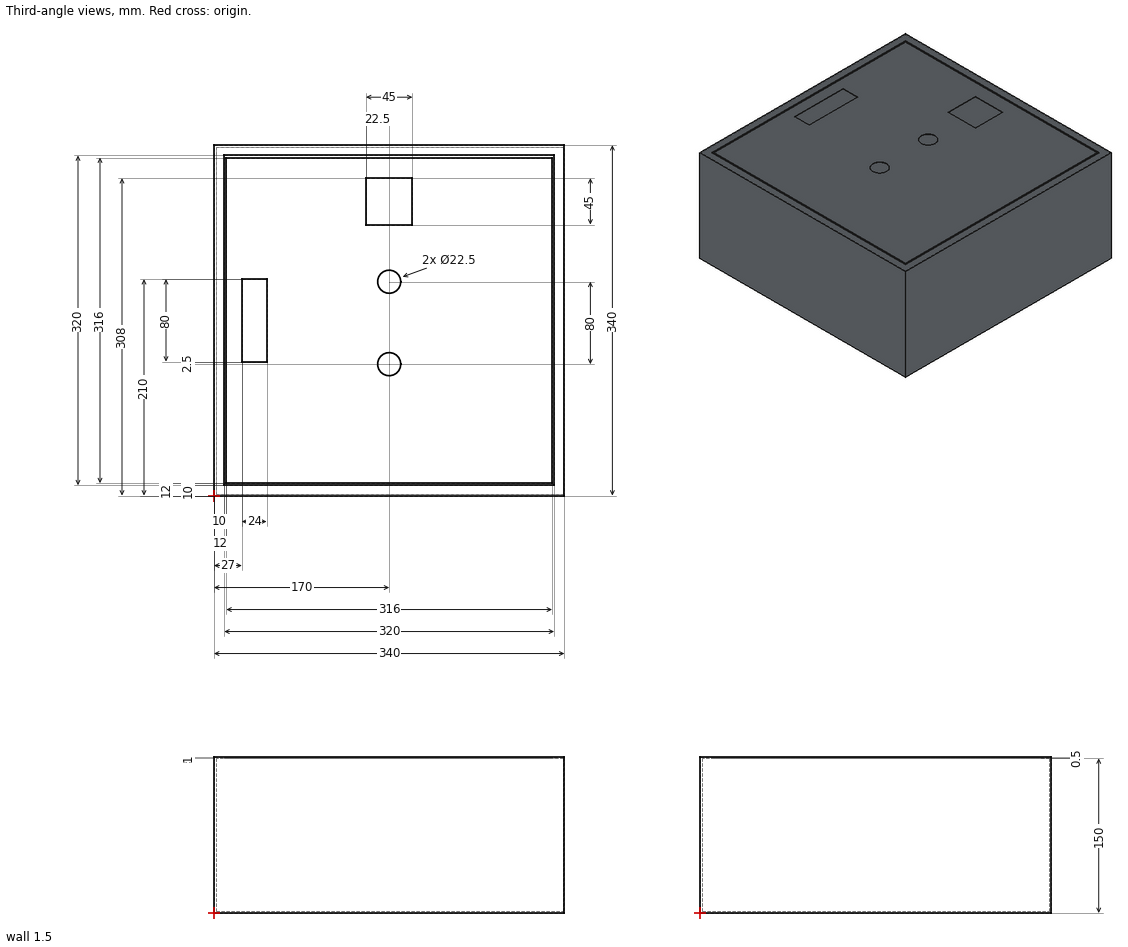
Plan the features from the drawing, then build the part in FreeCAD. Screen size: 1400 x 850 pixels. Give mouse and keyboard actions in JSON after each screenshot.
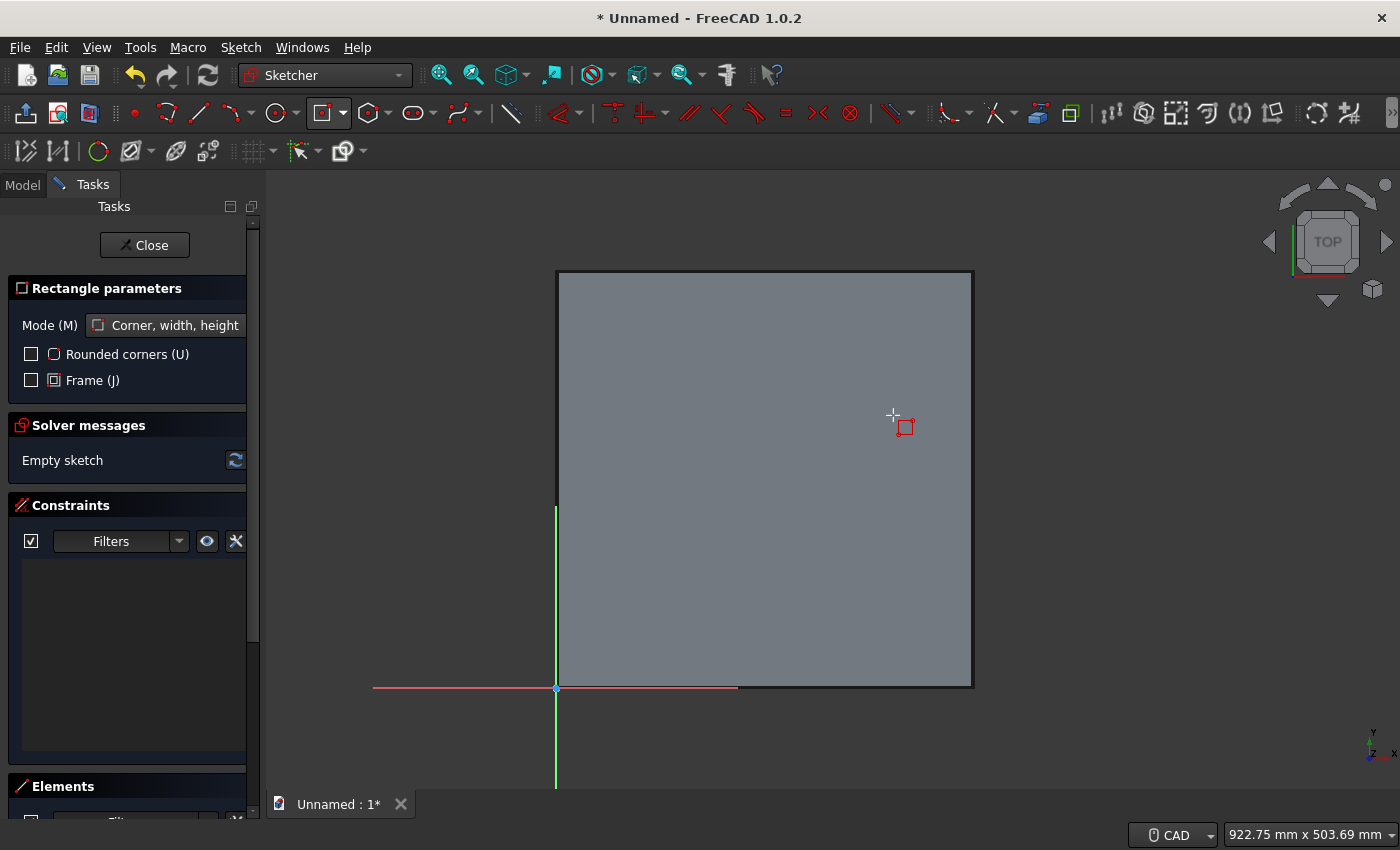
{"action": "left_click", "coordinate": [556, 688]}
{"action": "mouse_move", "coordinate": [974, 271]}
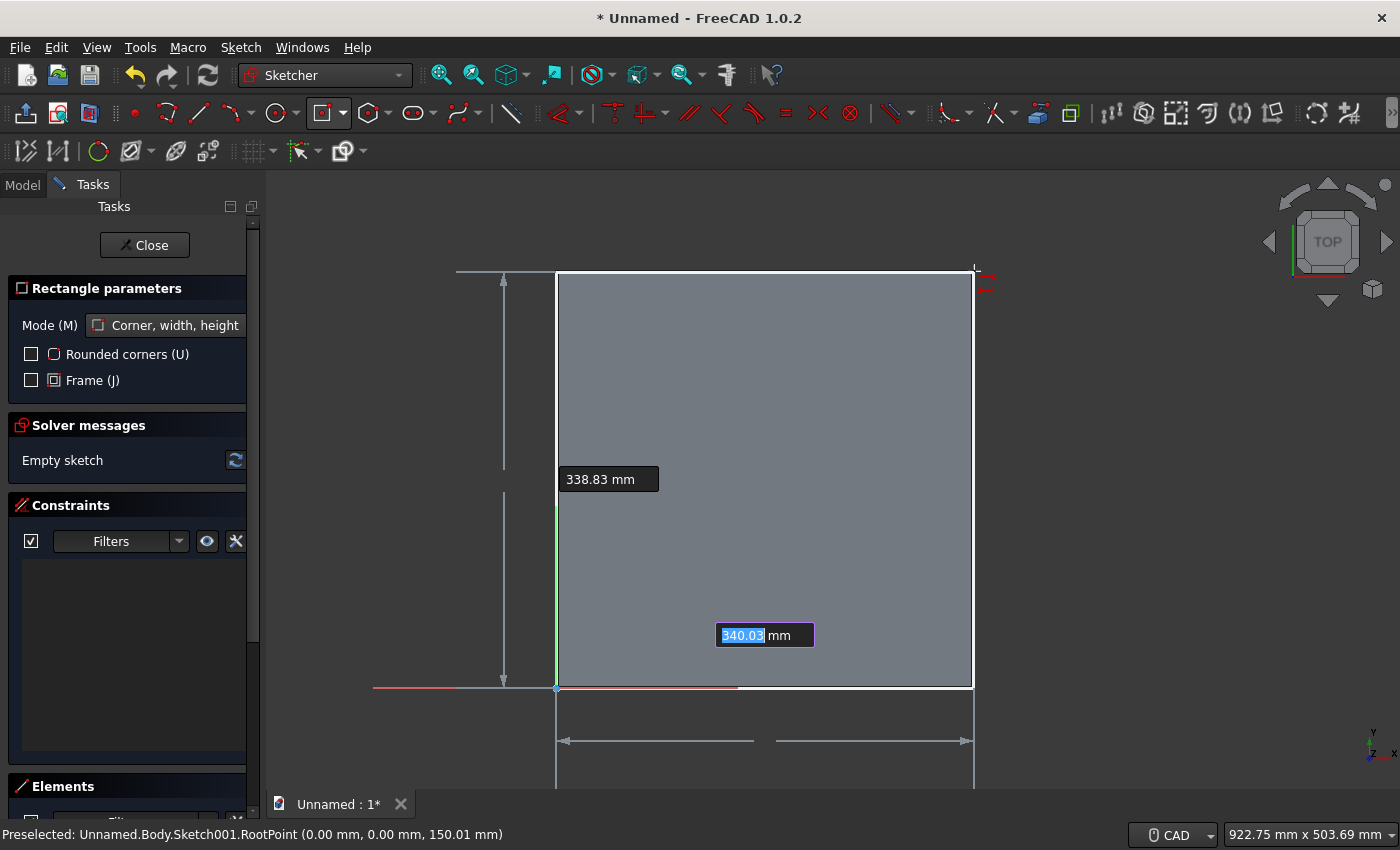
{"action": "type", "text": "340"}
{"action": "key", "text": "Tab"}
{"action": "type", "text": "340"}
{"action": "key", "text": "Return"}
{"action": "key", "text": "Escape"}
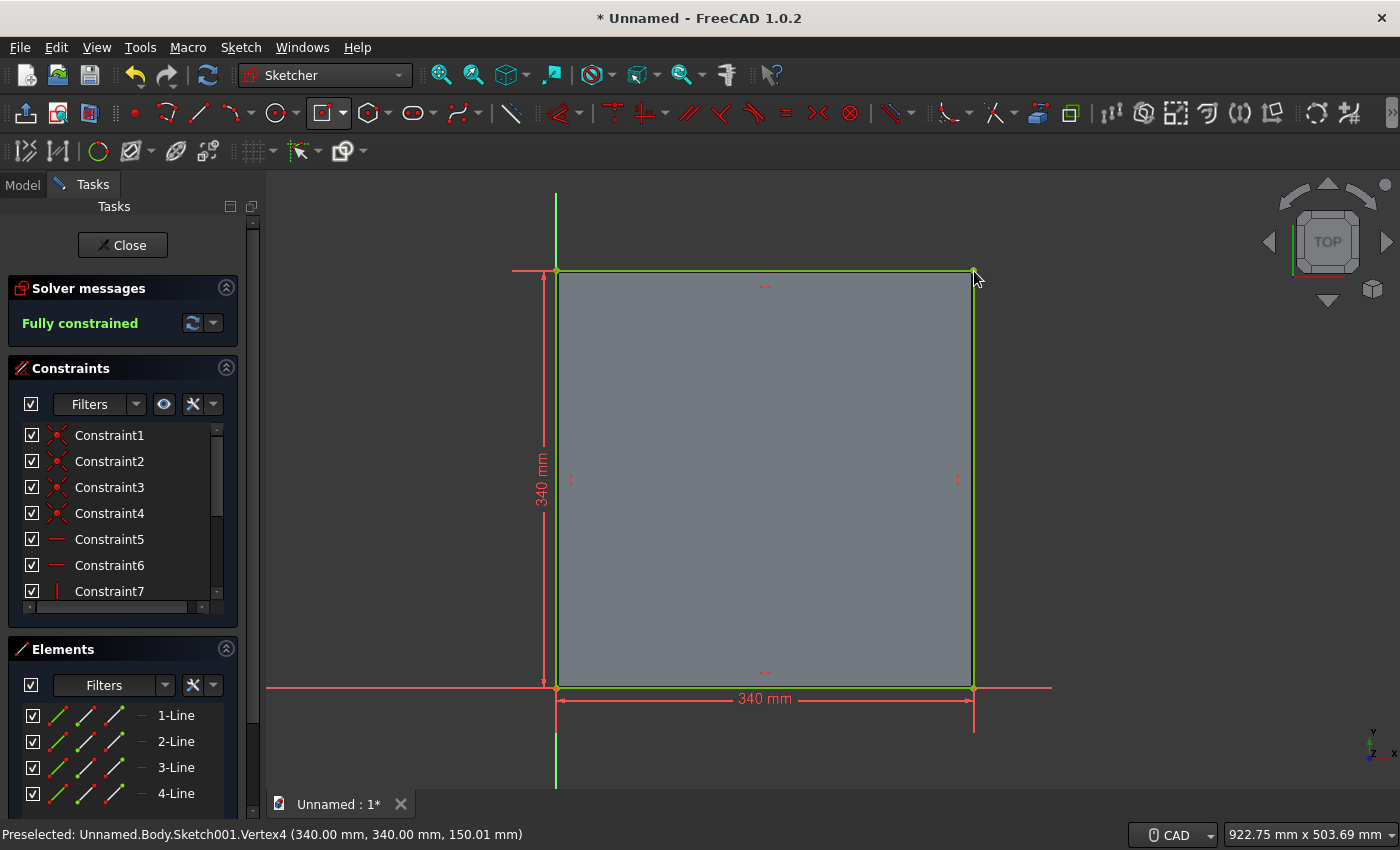
{"action": "left_click", "coordinate": [123, 245]}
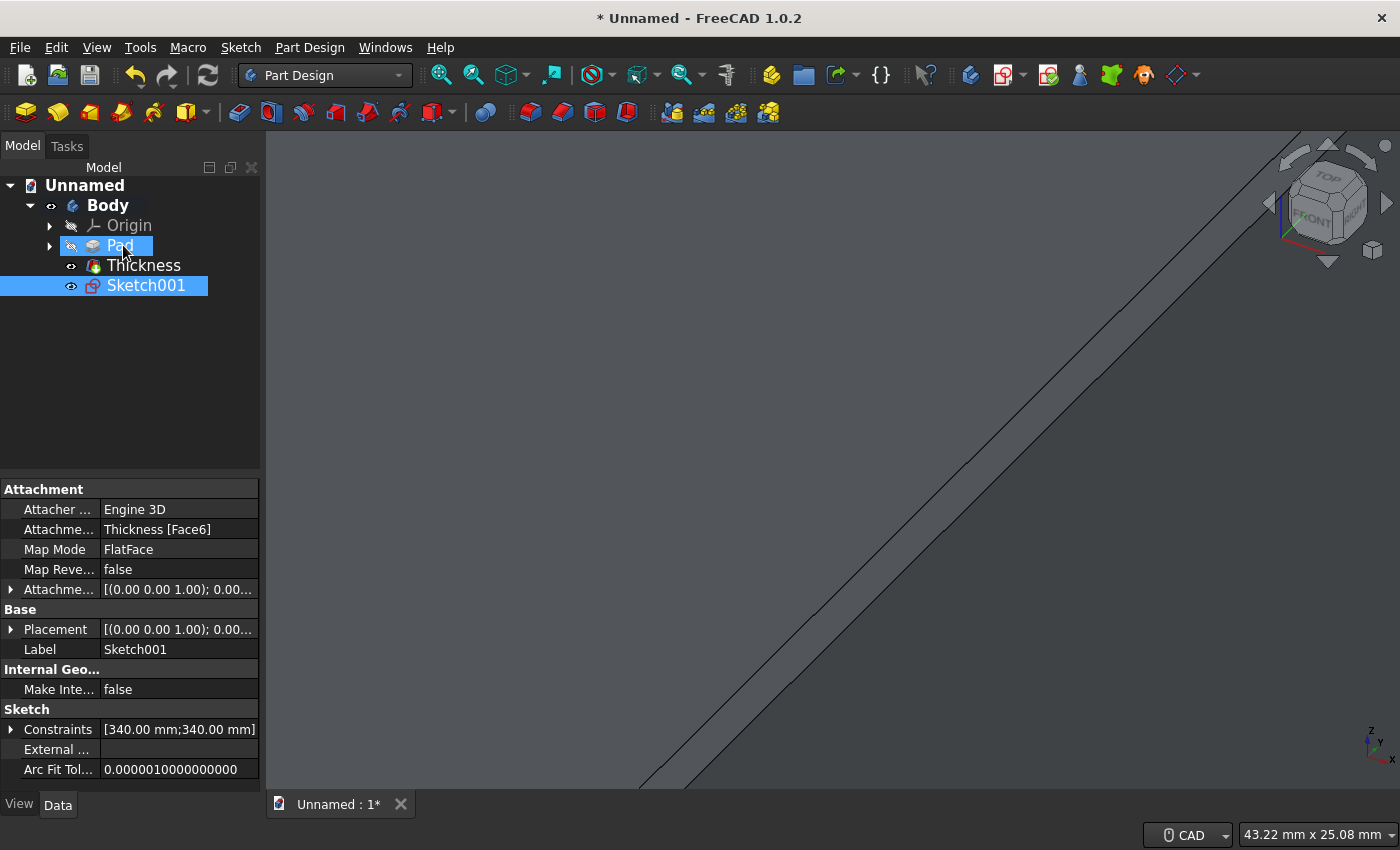
{"action": "left_click", "coordinate": [26, 112]}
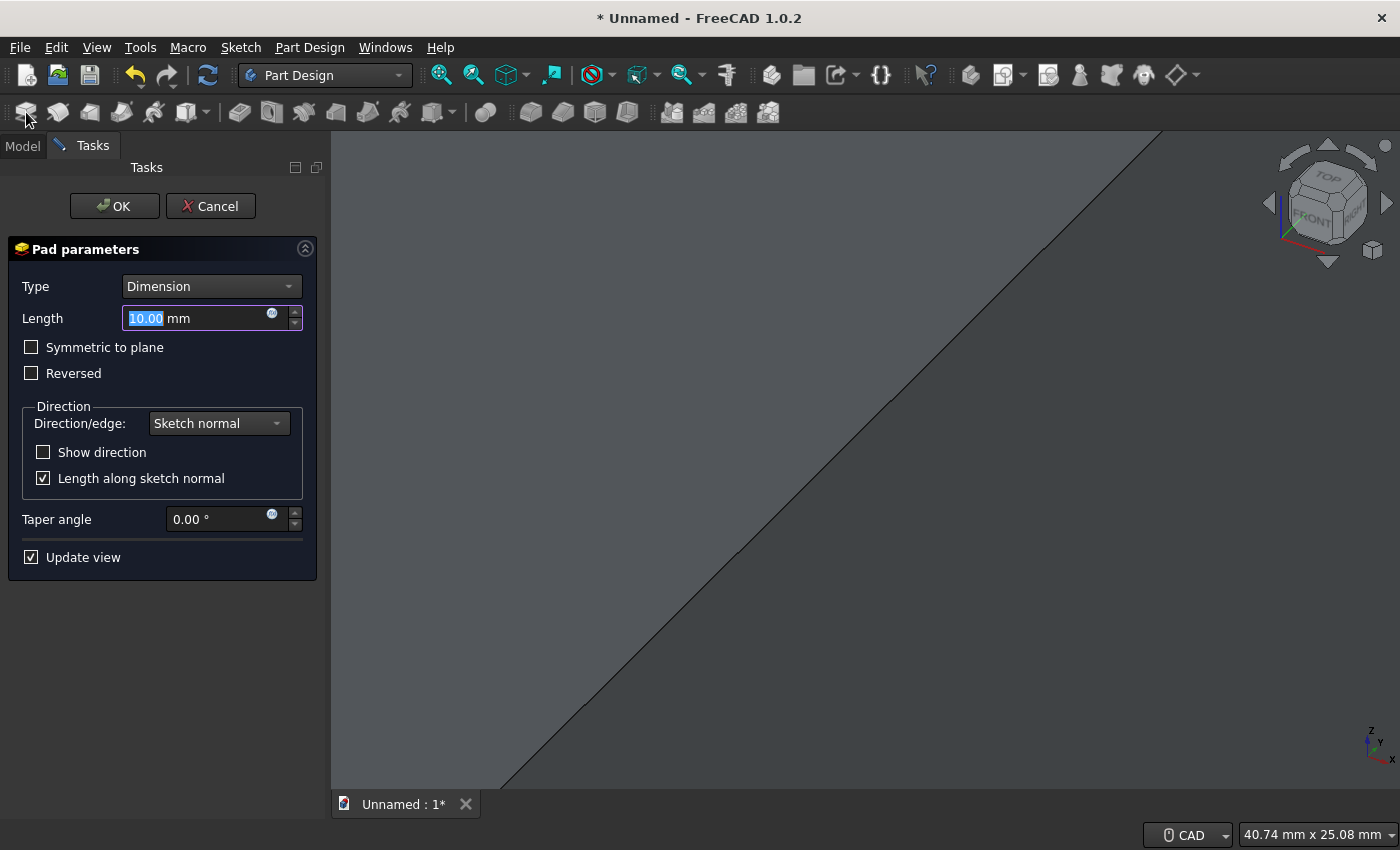
{"action": "type", "text": "1"}
{"action": "key", "text": "Tab"}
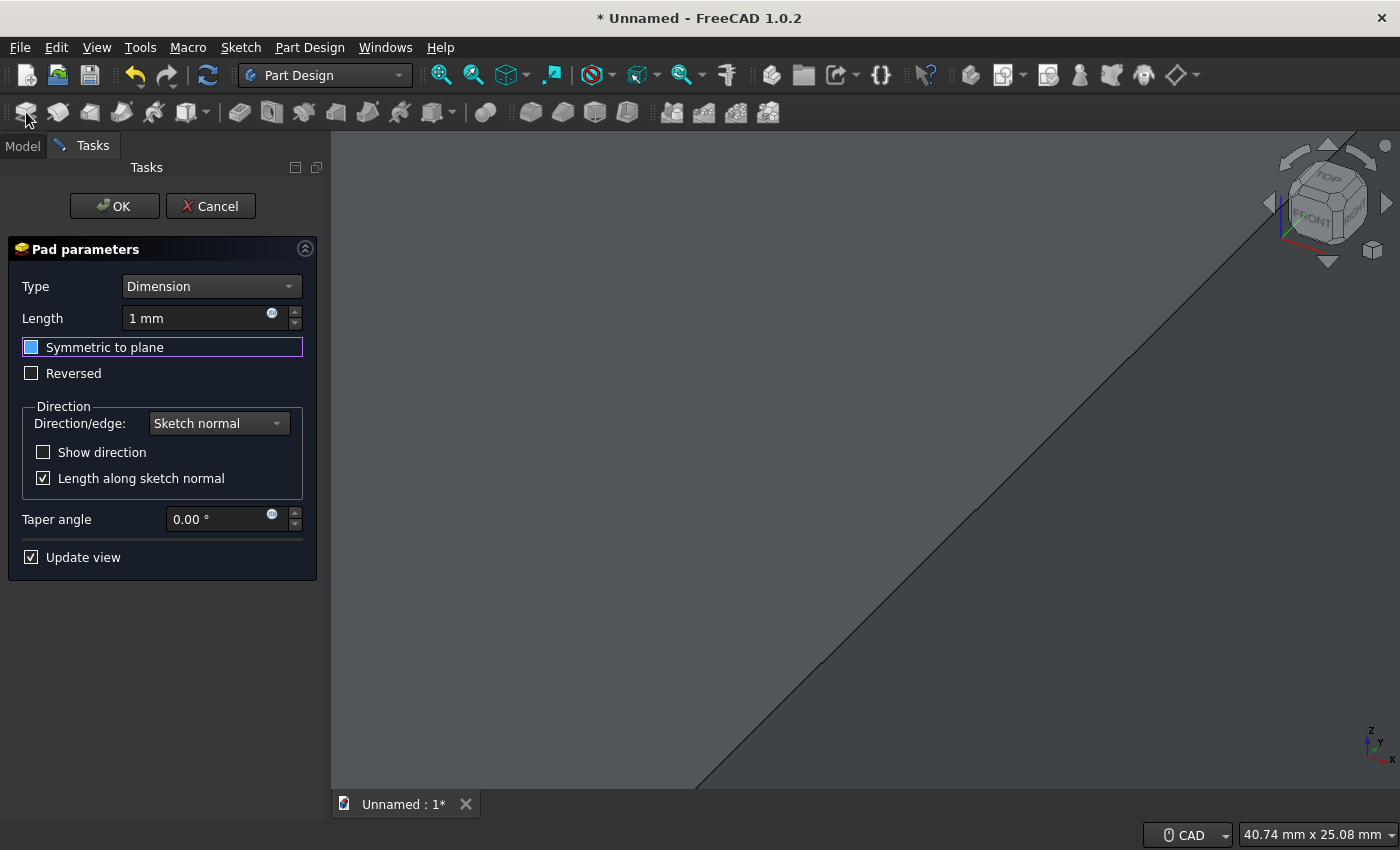
{"action": "left_click", "coordinate": [115, 206]}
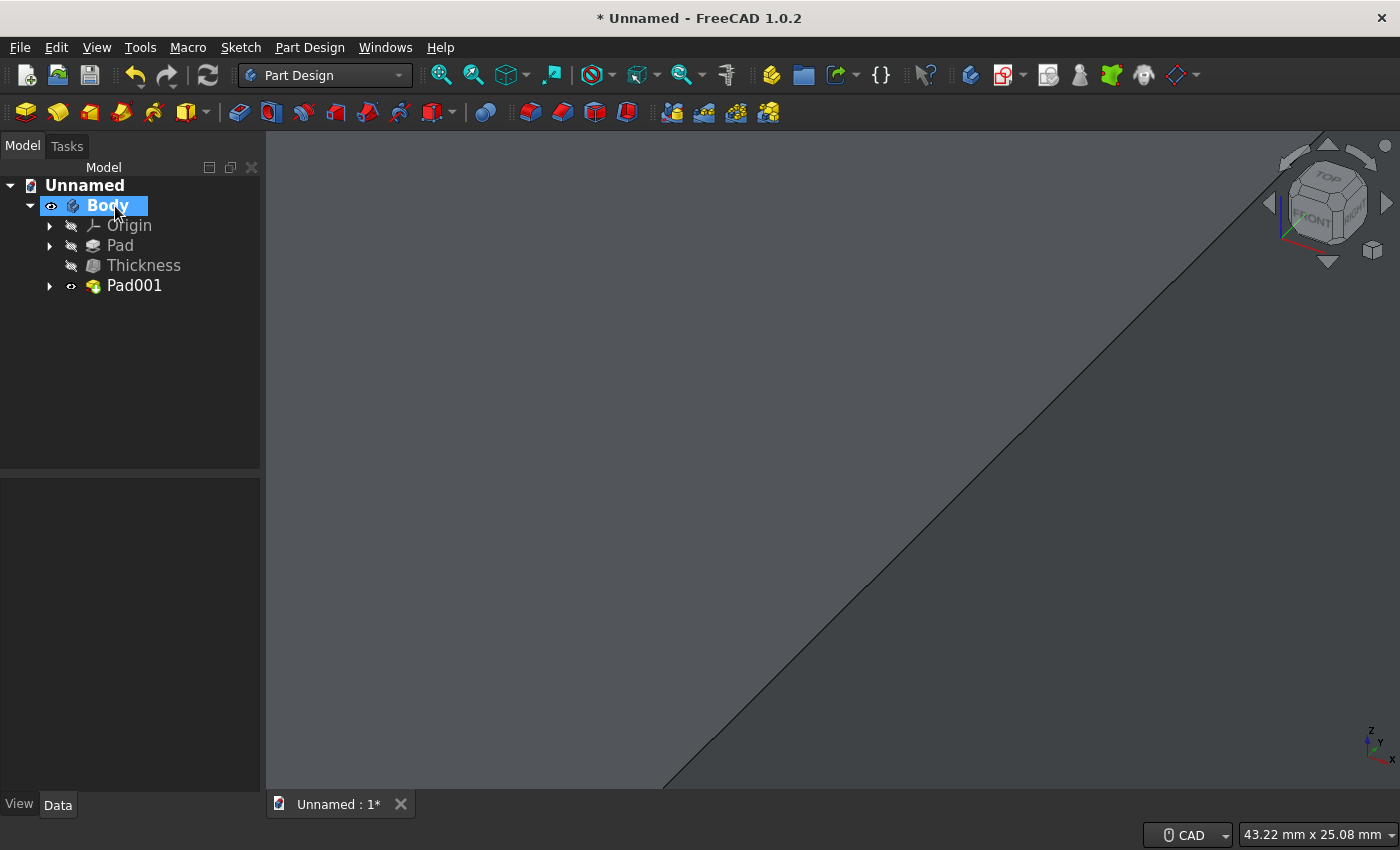
{"action": "key", "text": "v f"}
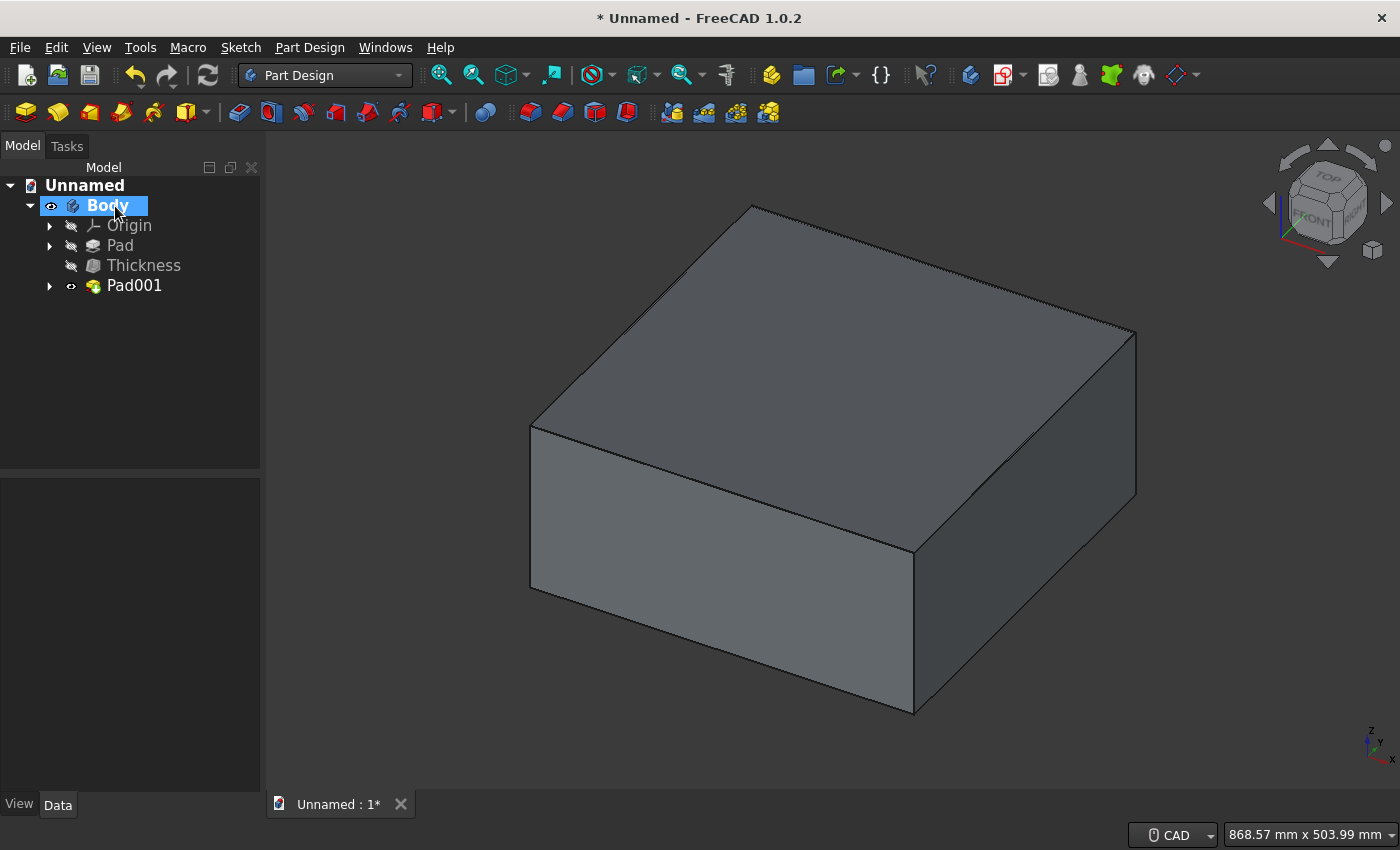
{"action": "left_click", "coordinate": [833, 378]}